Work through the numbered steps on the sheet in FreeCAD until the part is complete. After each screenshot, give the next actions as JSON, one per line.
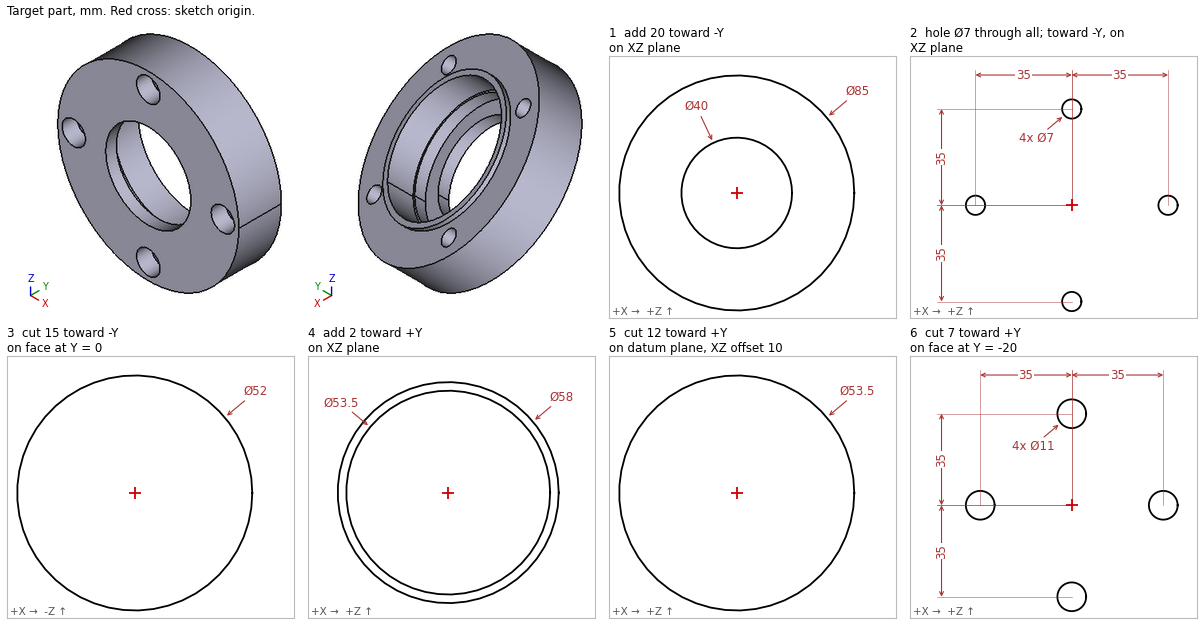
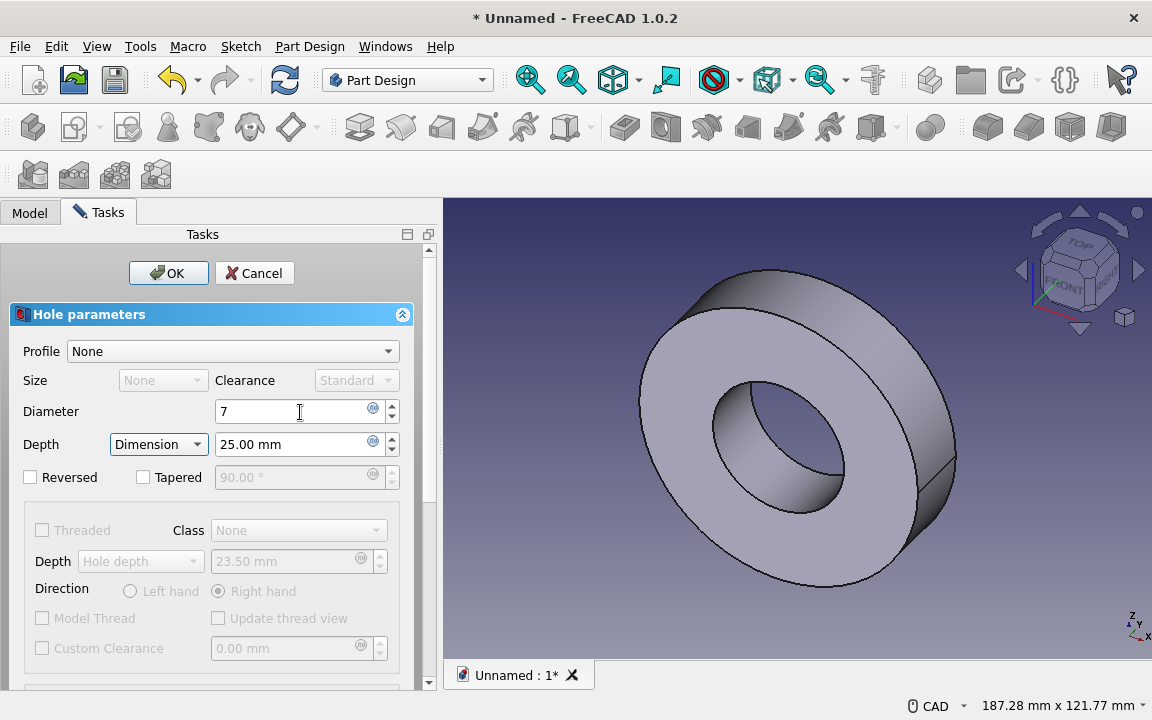
{"action": "left_click", "coordinate": [160, 444]}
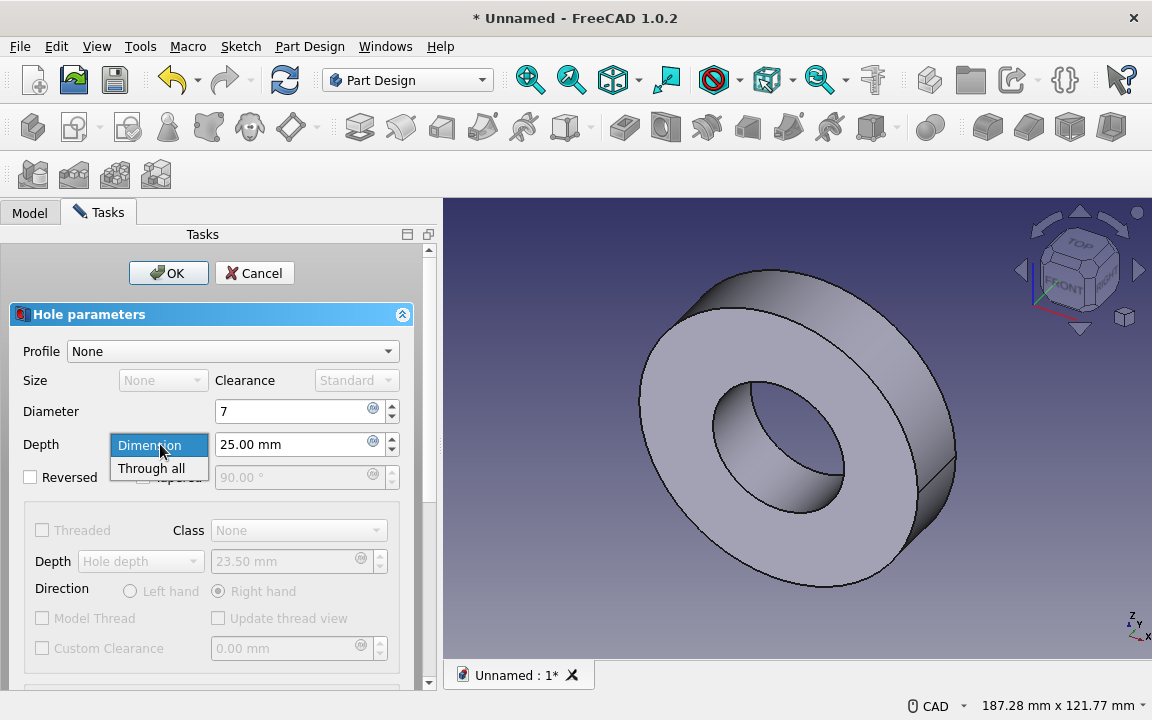
{"action": "left_click", "coordinate": [158, 468]}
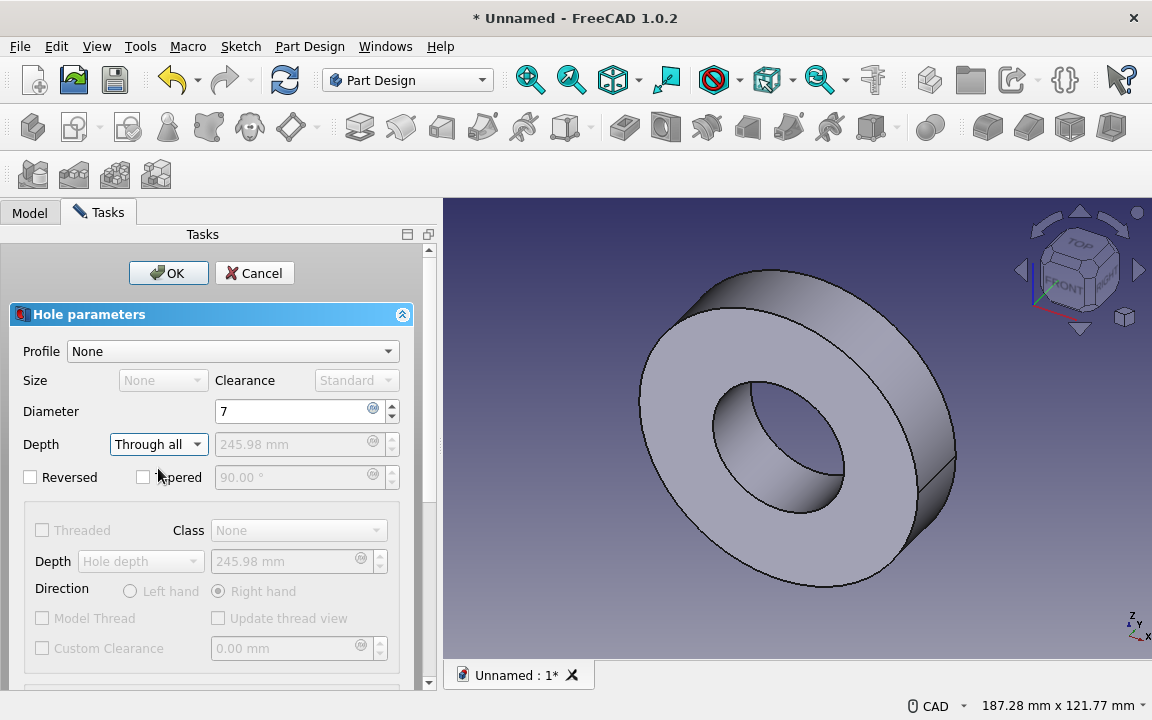
{"action": "left_click", "coordinate": [31, 477]}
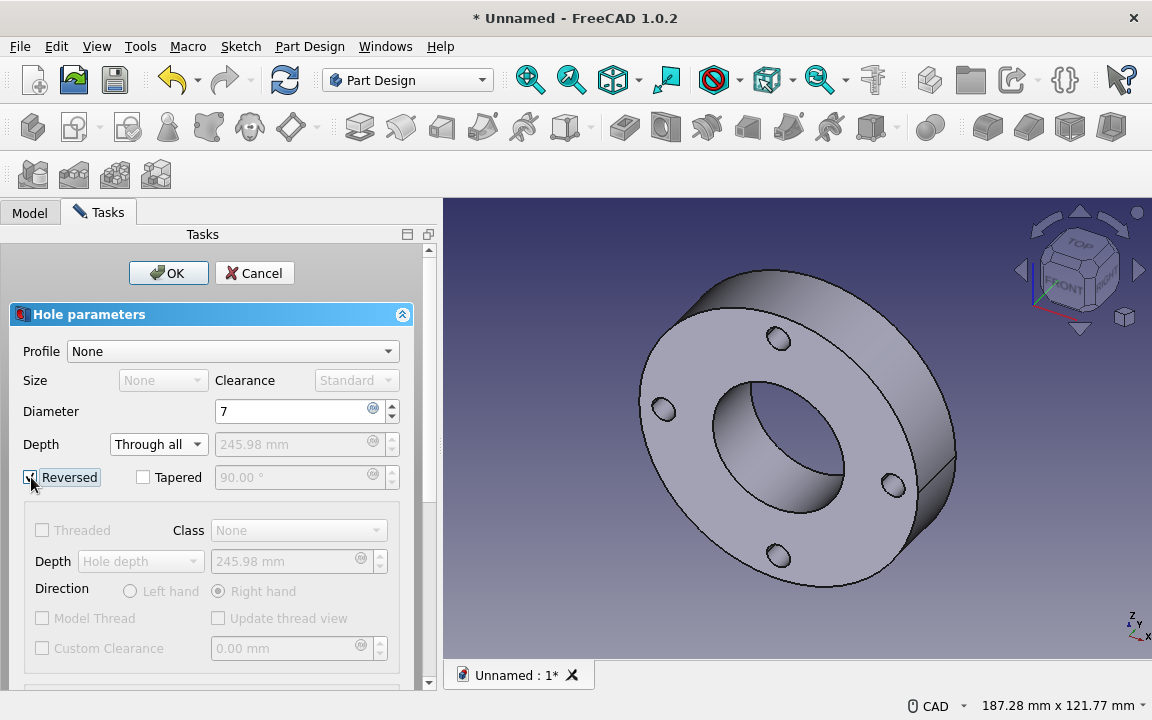
{"action": "left_click", "coordinate": [169, 273]}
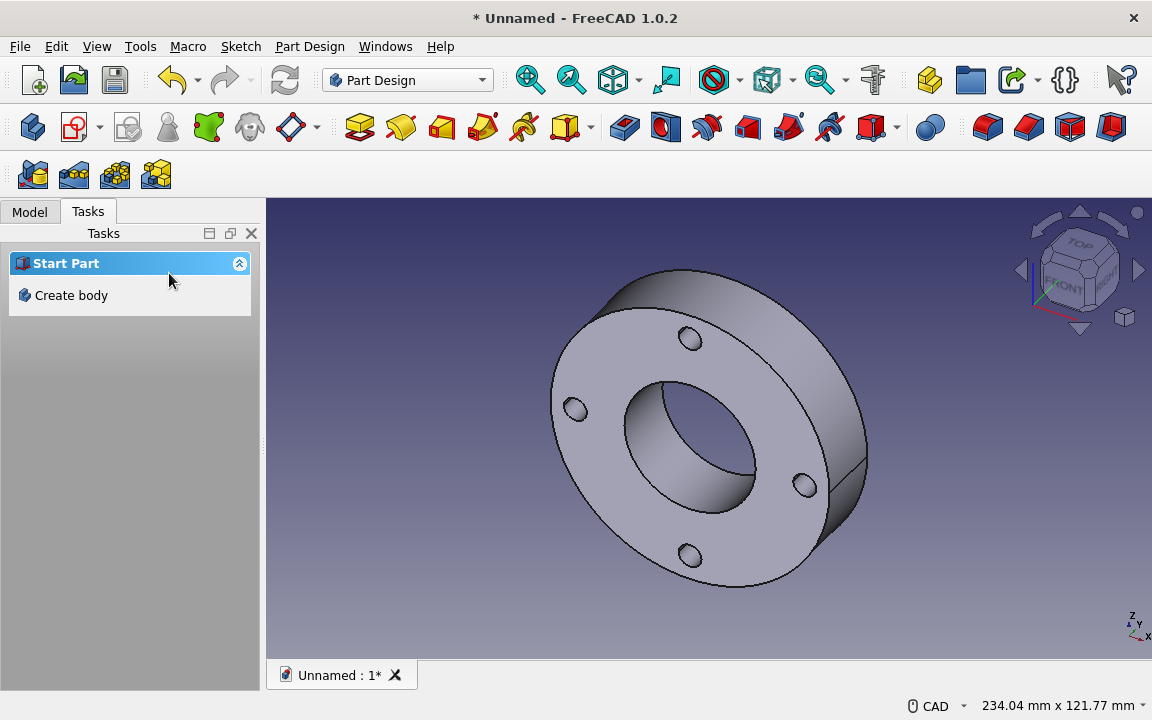
{"action": "key", "text": "4"}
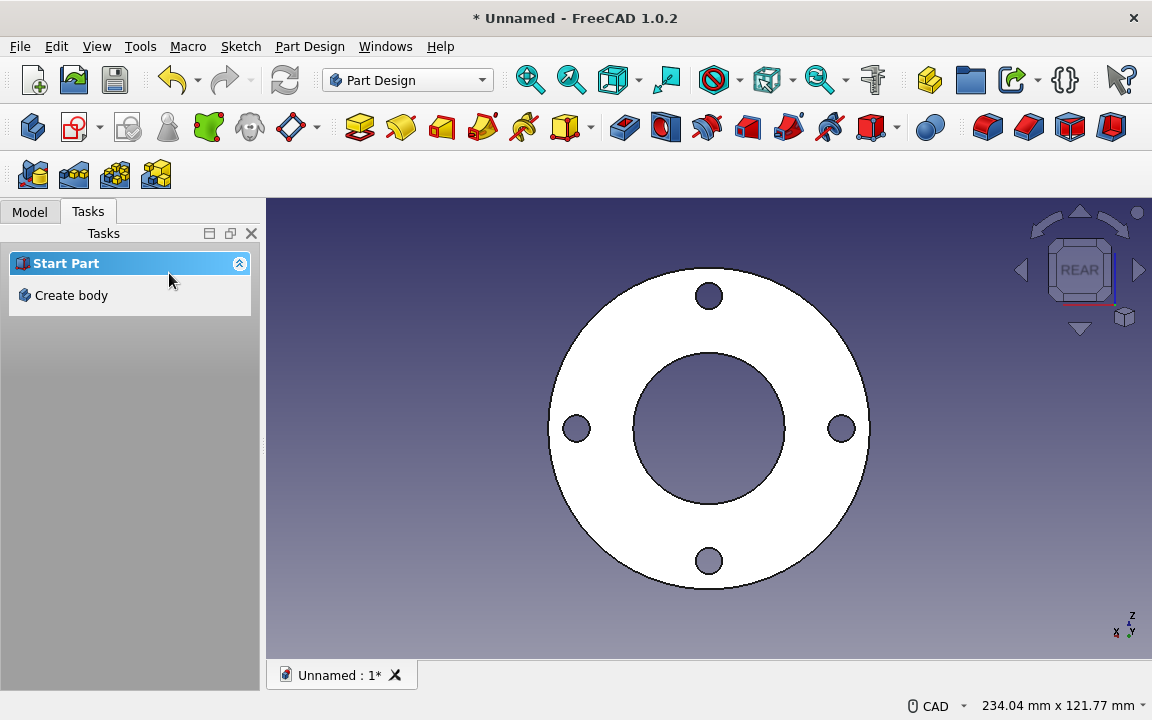
{"action": "left_click", "coordinate": [617, 519]}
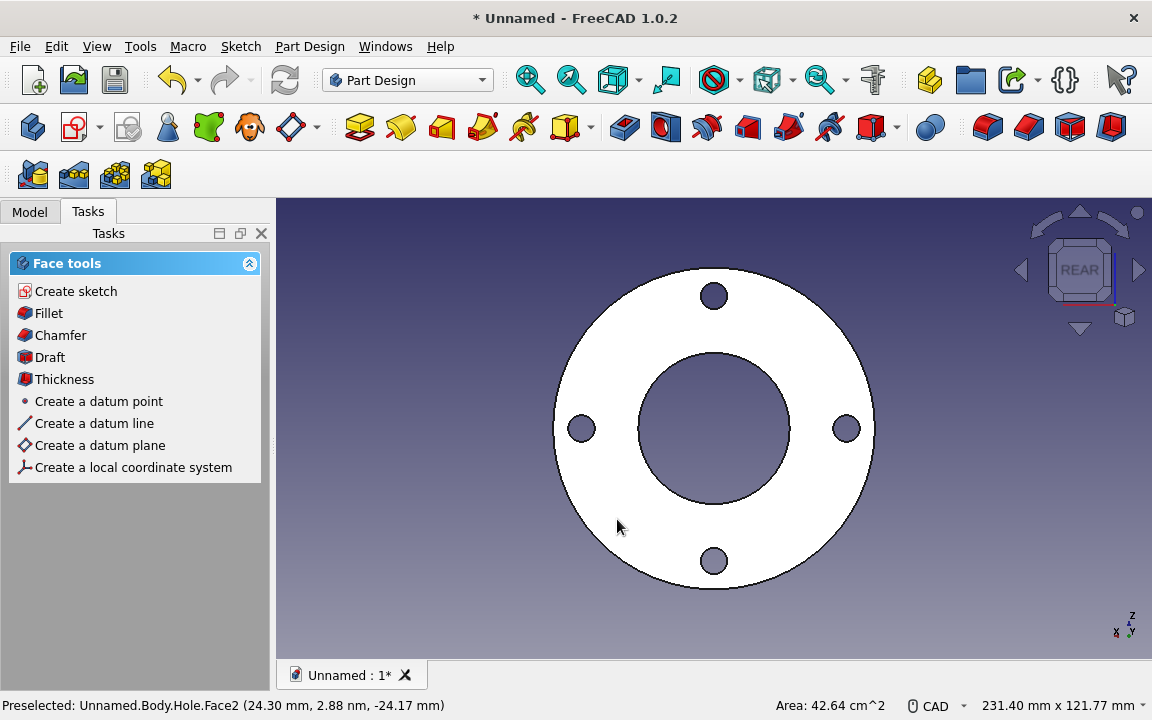
{"action": "left_click", "coordinate": [74, 128]}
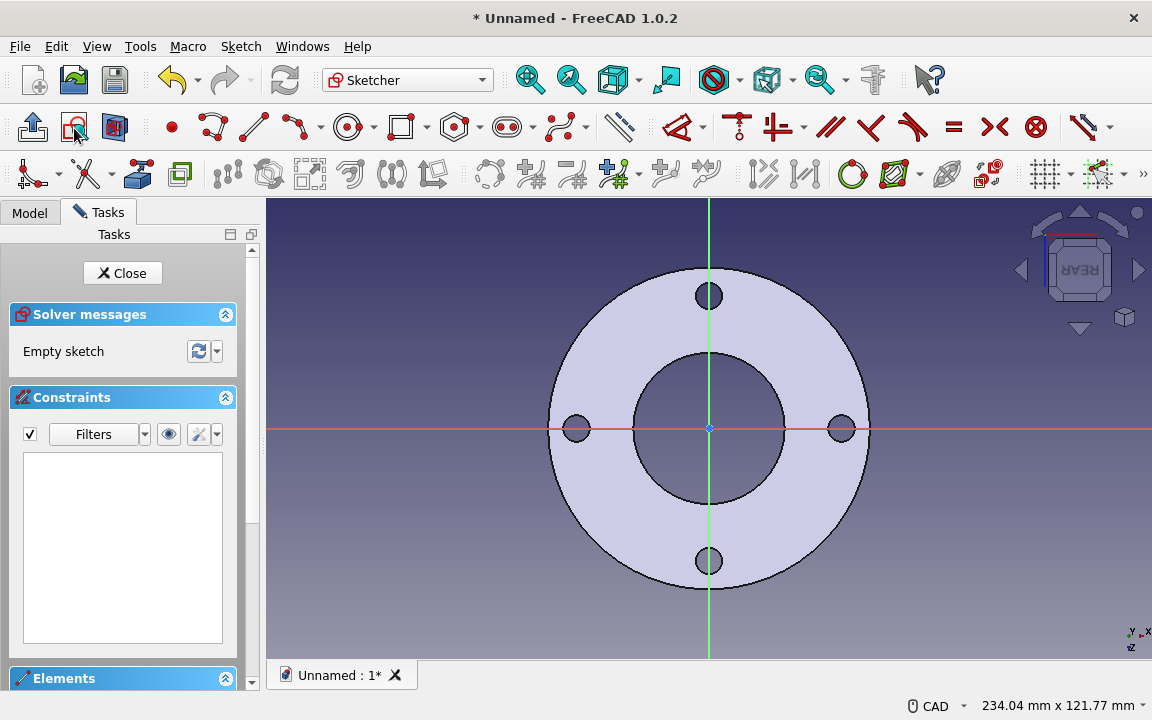
{"action": "scroll", "coordinate": [848, 429], "scroll_direction": "up", "scroll_amount": 2}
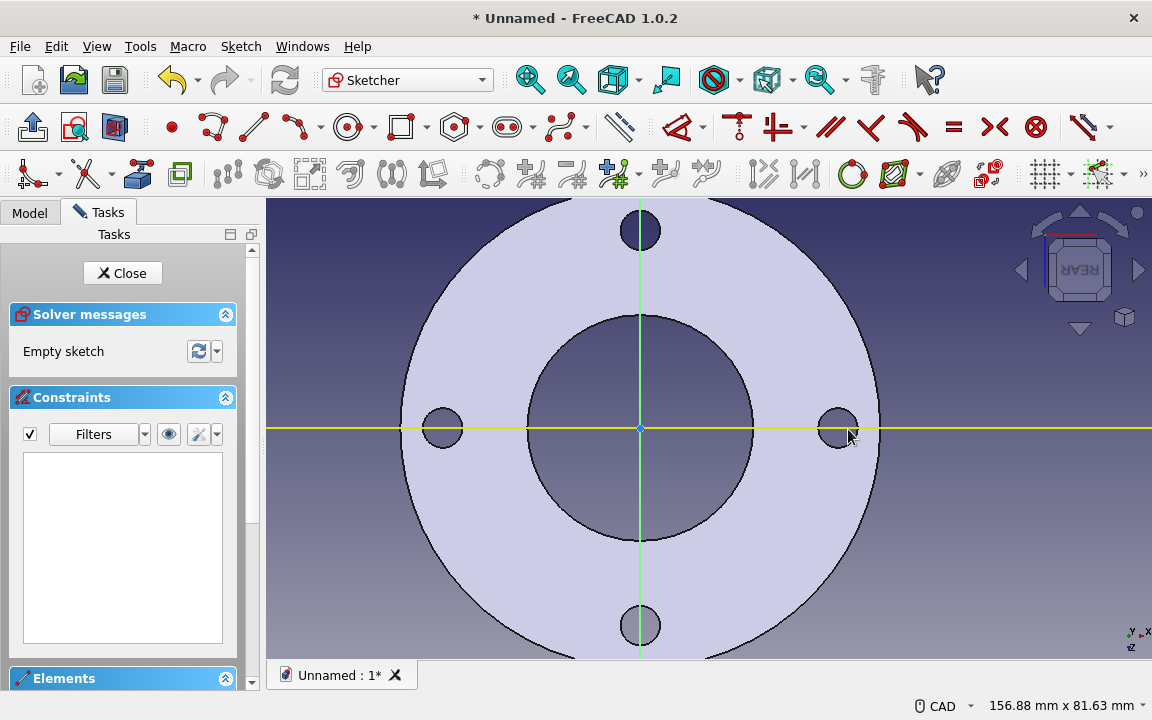
{"action": "left_click", "coordinate": [348, 128]}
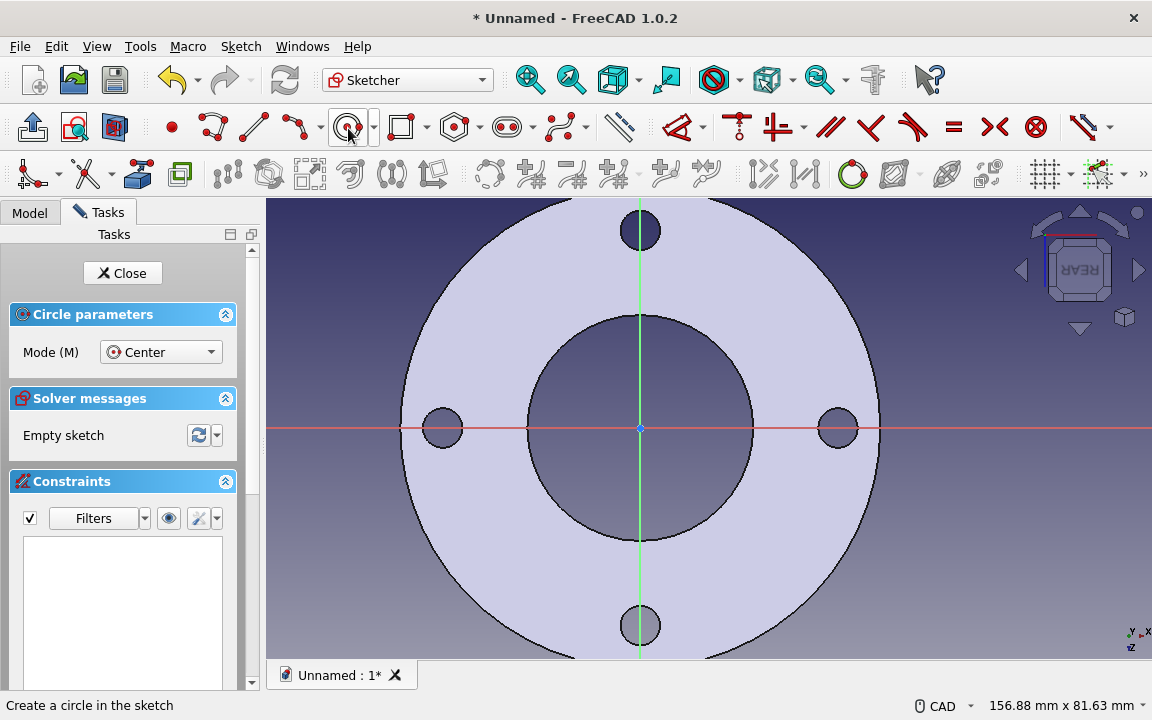
{"action": "left_click", "coordinate": [640, 428]}
{"action": "mouse_move", "coordinate": [744, 324]}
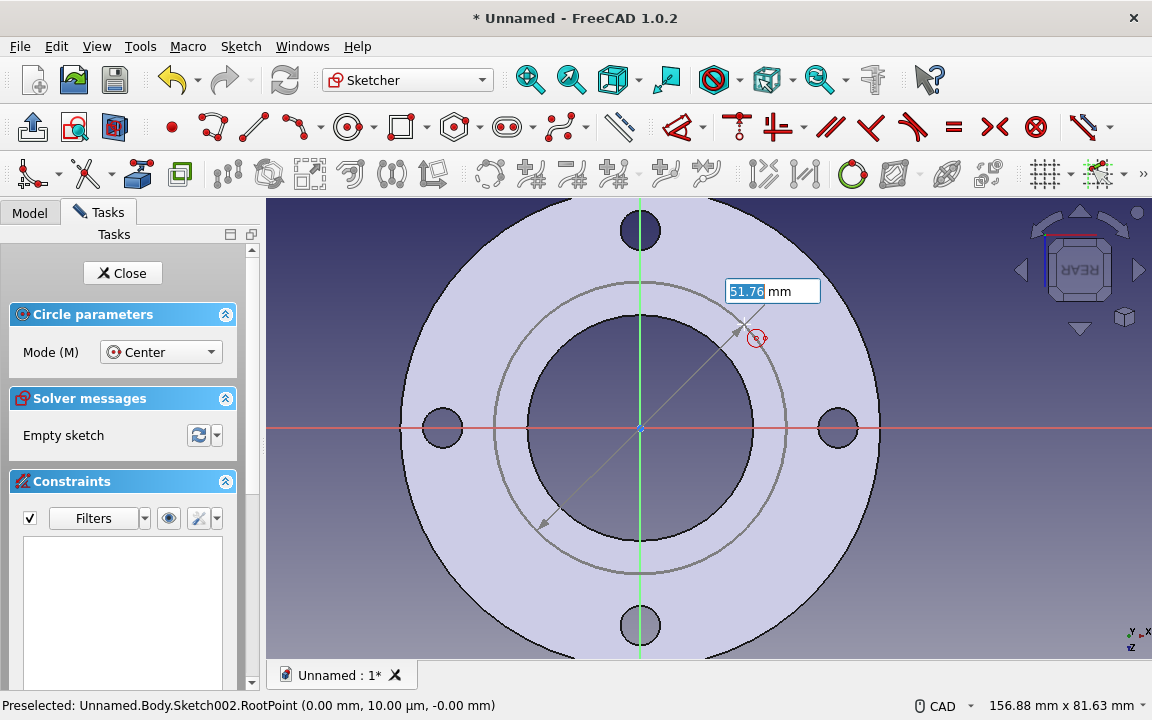
{"action": "type", "text": "52"}
{"action": "key", "text": "Return"}
{"action": "key", "text": "Escape"}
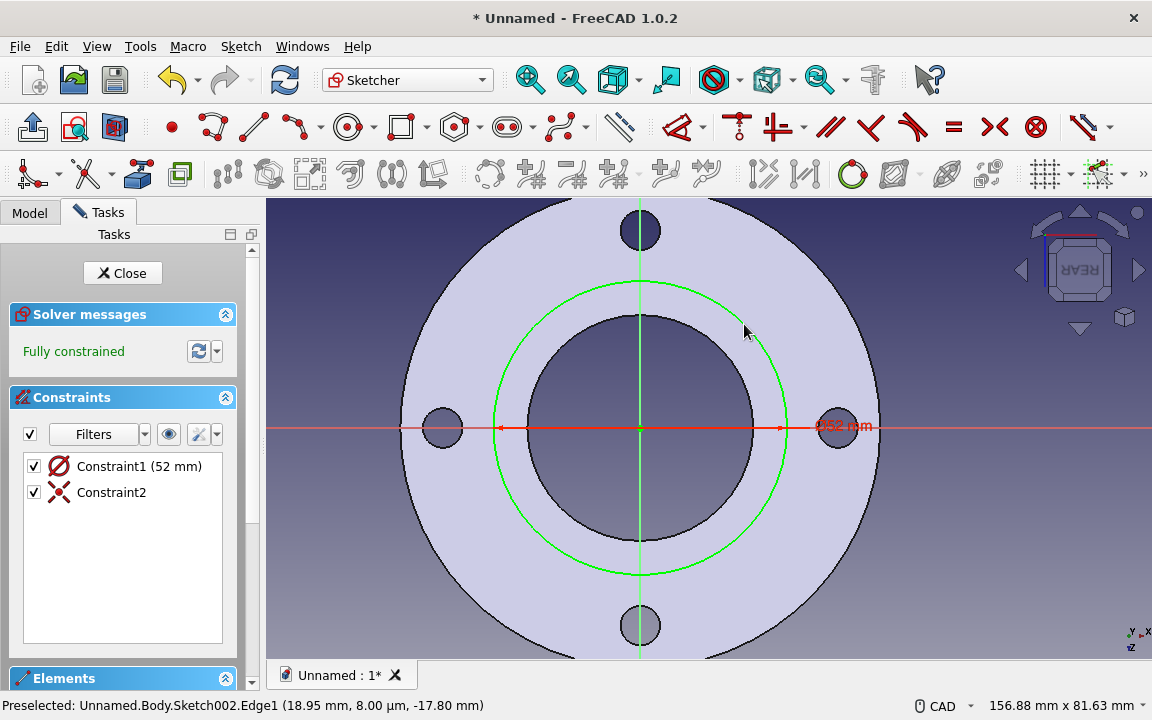
{"action": "left_click", "coordinate": [123, 273]}